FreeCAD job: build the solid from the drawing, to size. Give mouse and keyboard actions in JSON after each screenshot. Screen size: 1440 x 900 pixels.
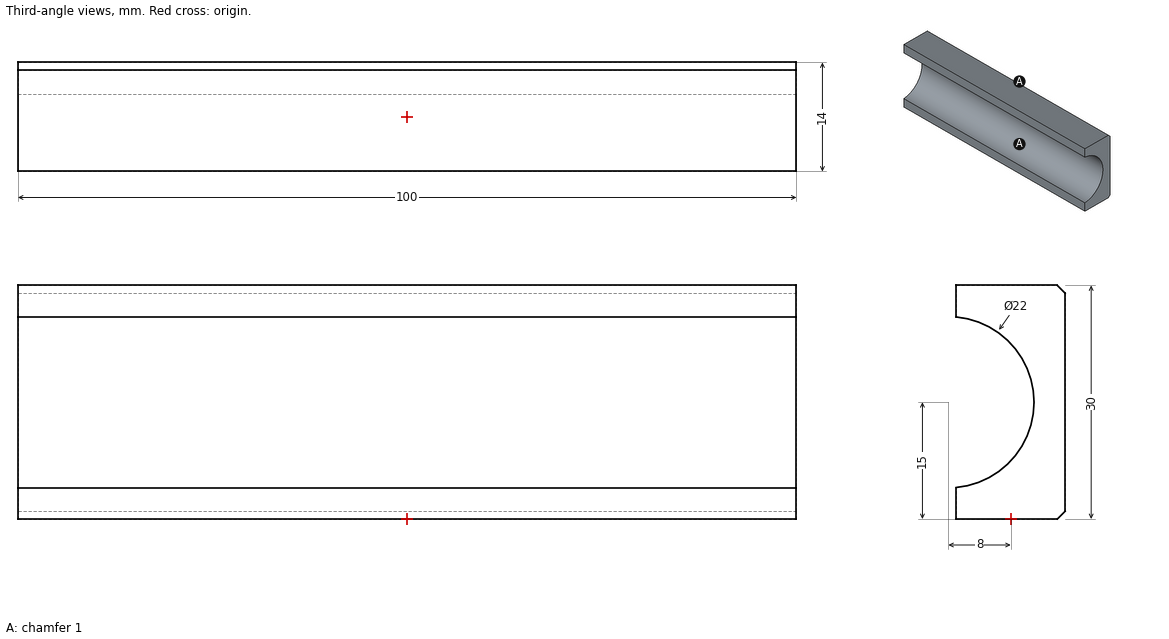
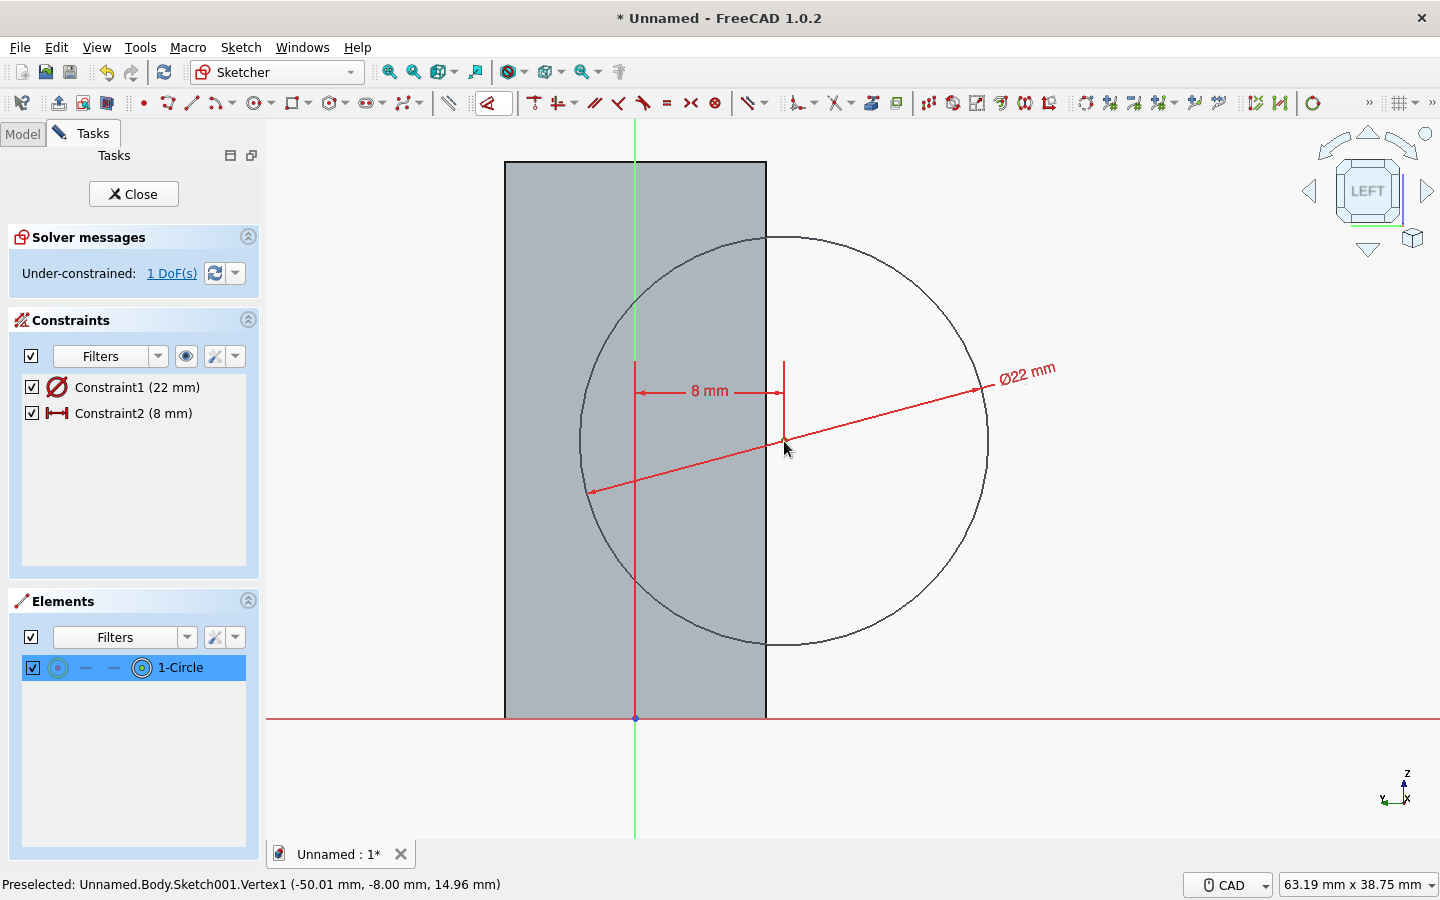
{"action": "key", "text": "i"}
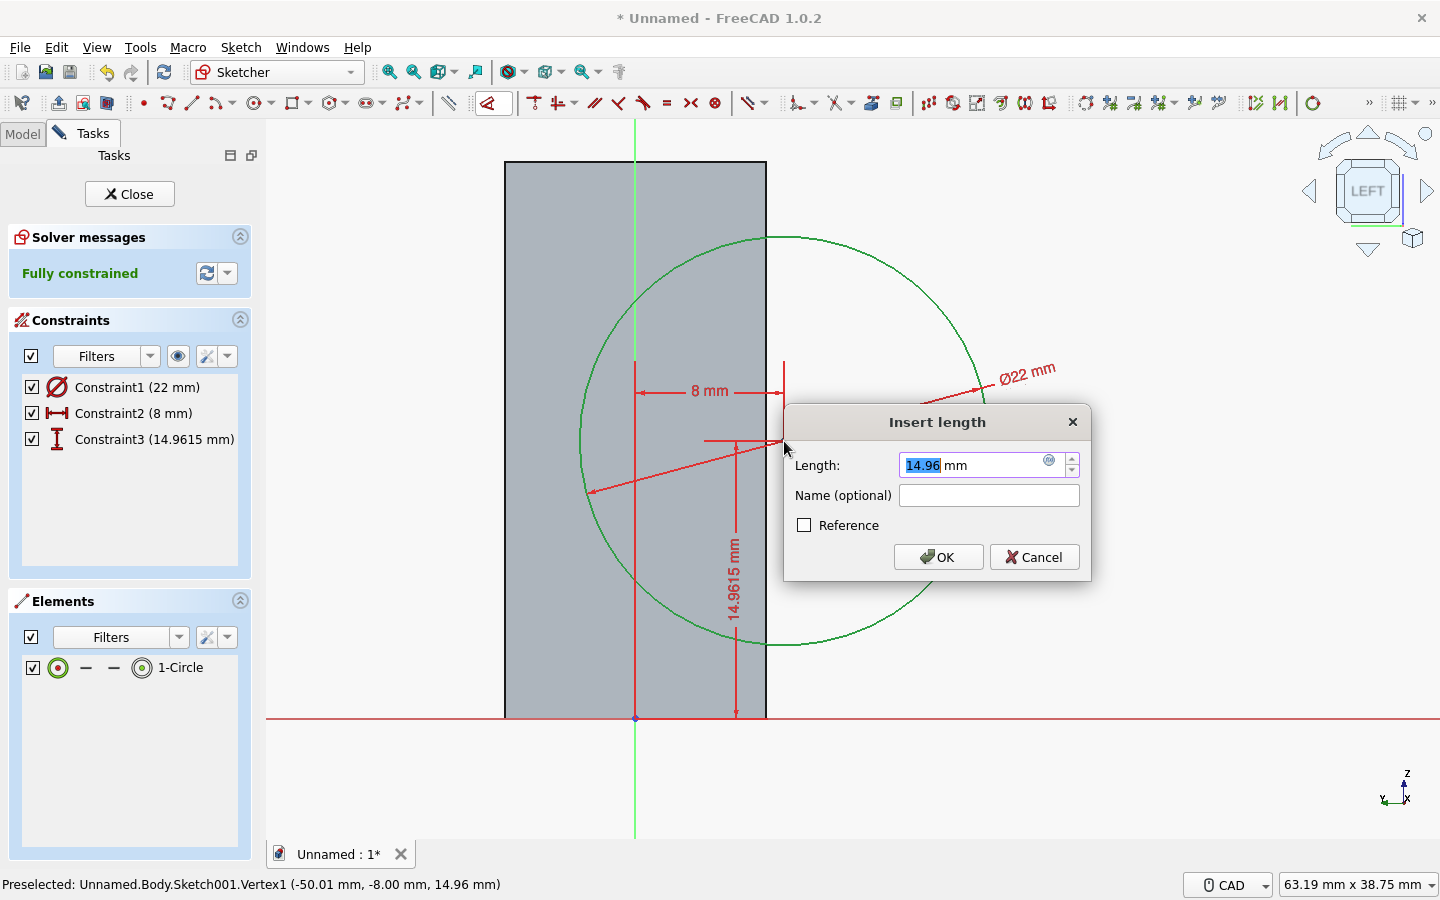
{"action": "type", "text": "15"}
{"action": "key", "text": "Return"}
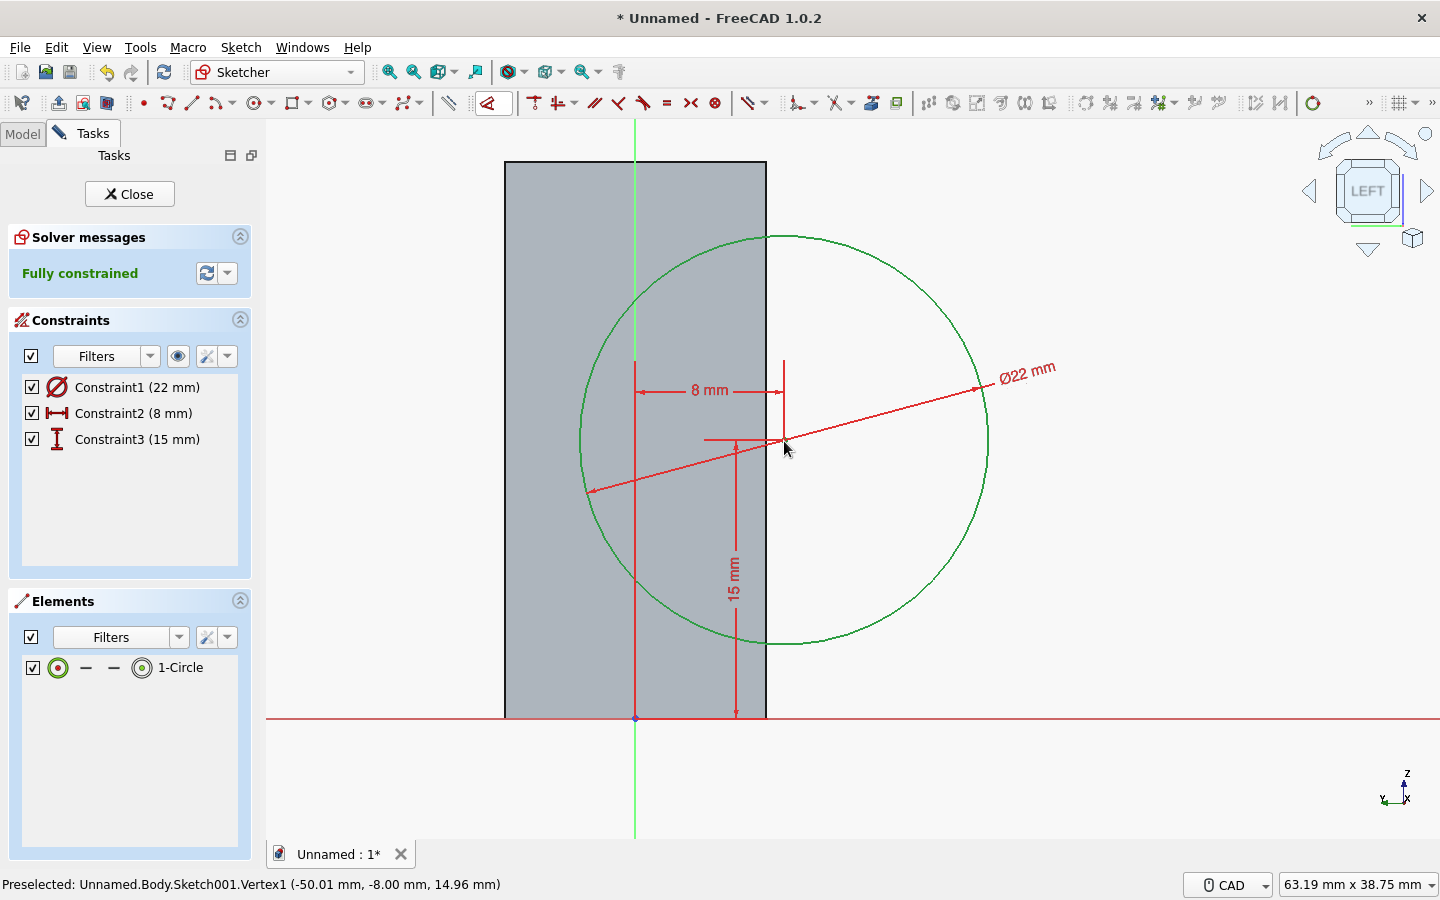
{"action": "left_click", "coordinate": [130, 194]}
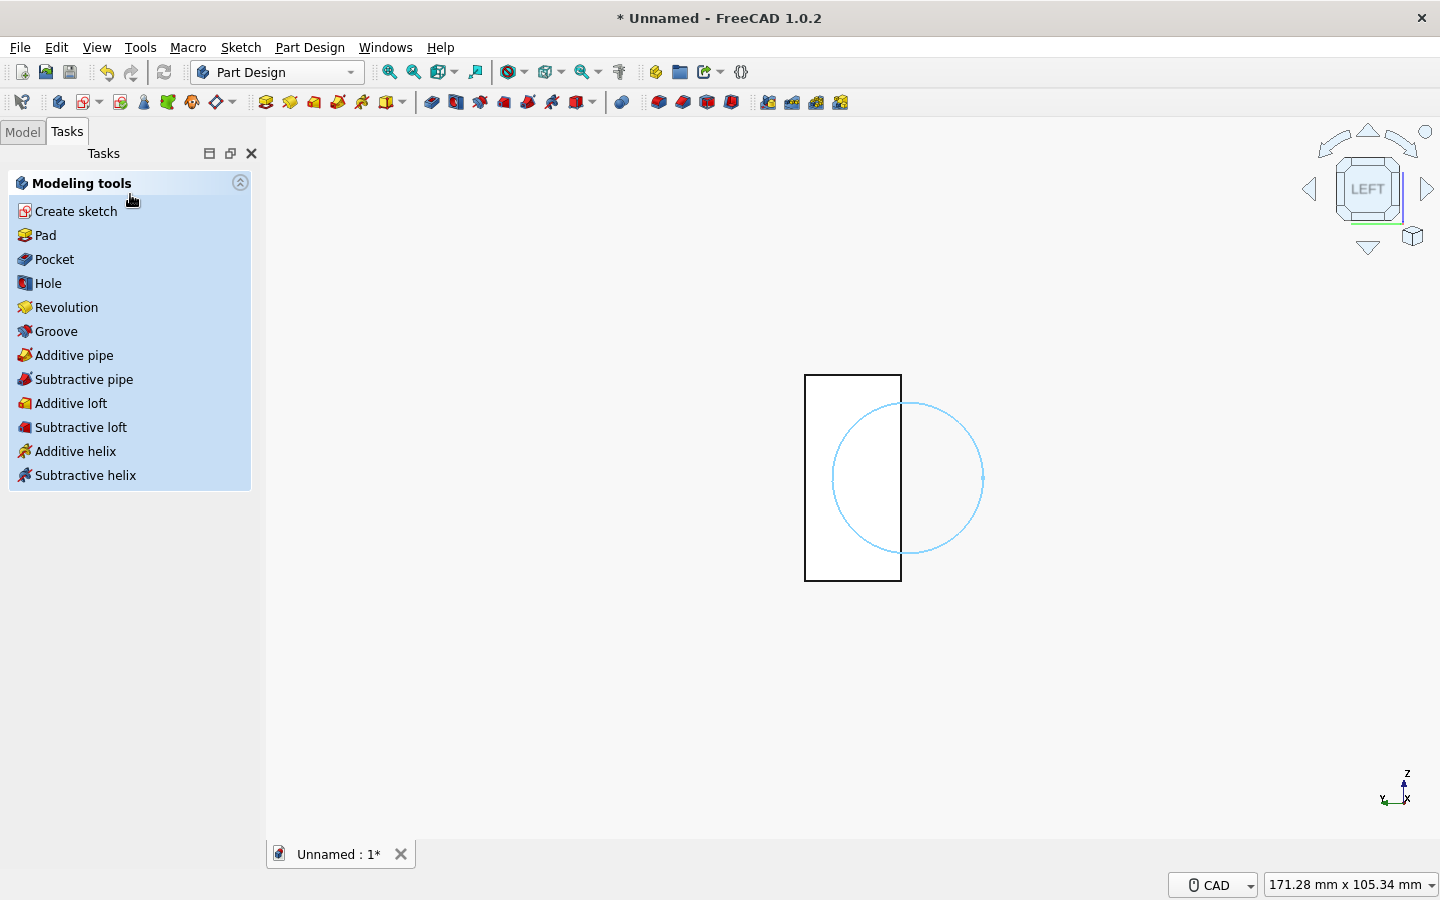
{"action": "left_click", "coordinate": [432, 102]}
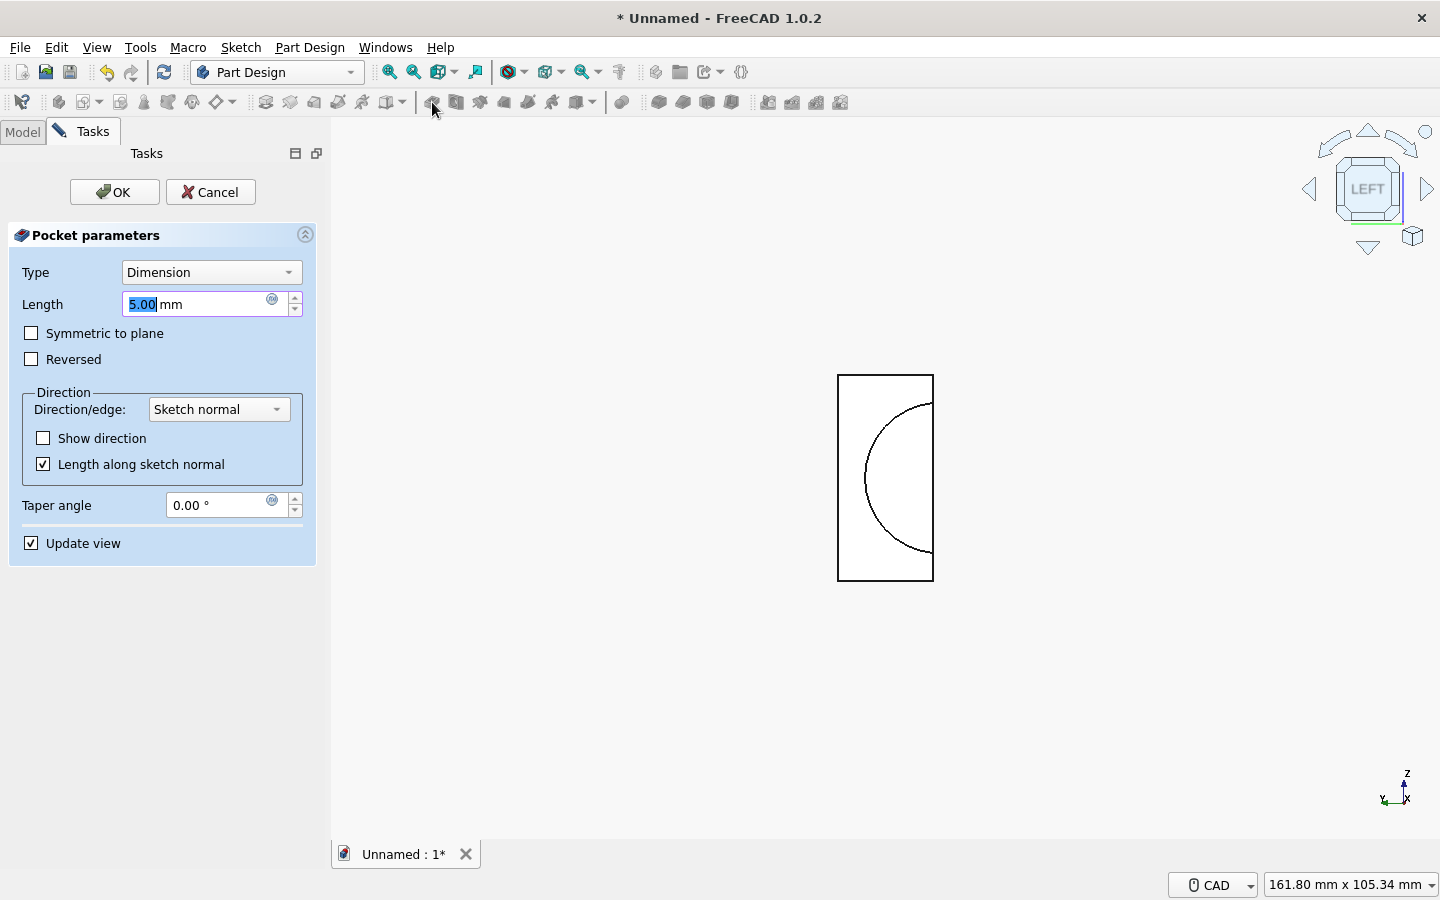
{"action": "left_click", "coordinate": [212, 272]}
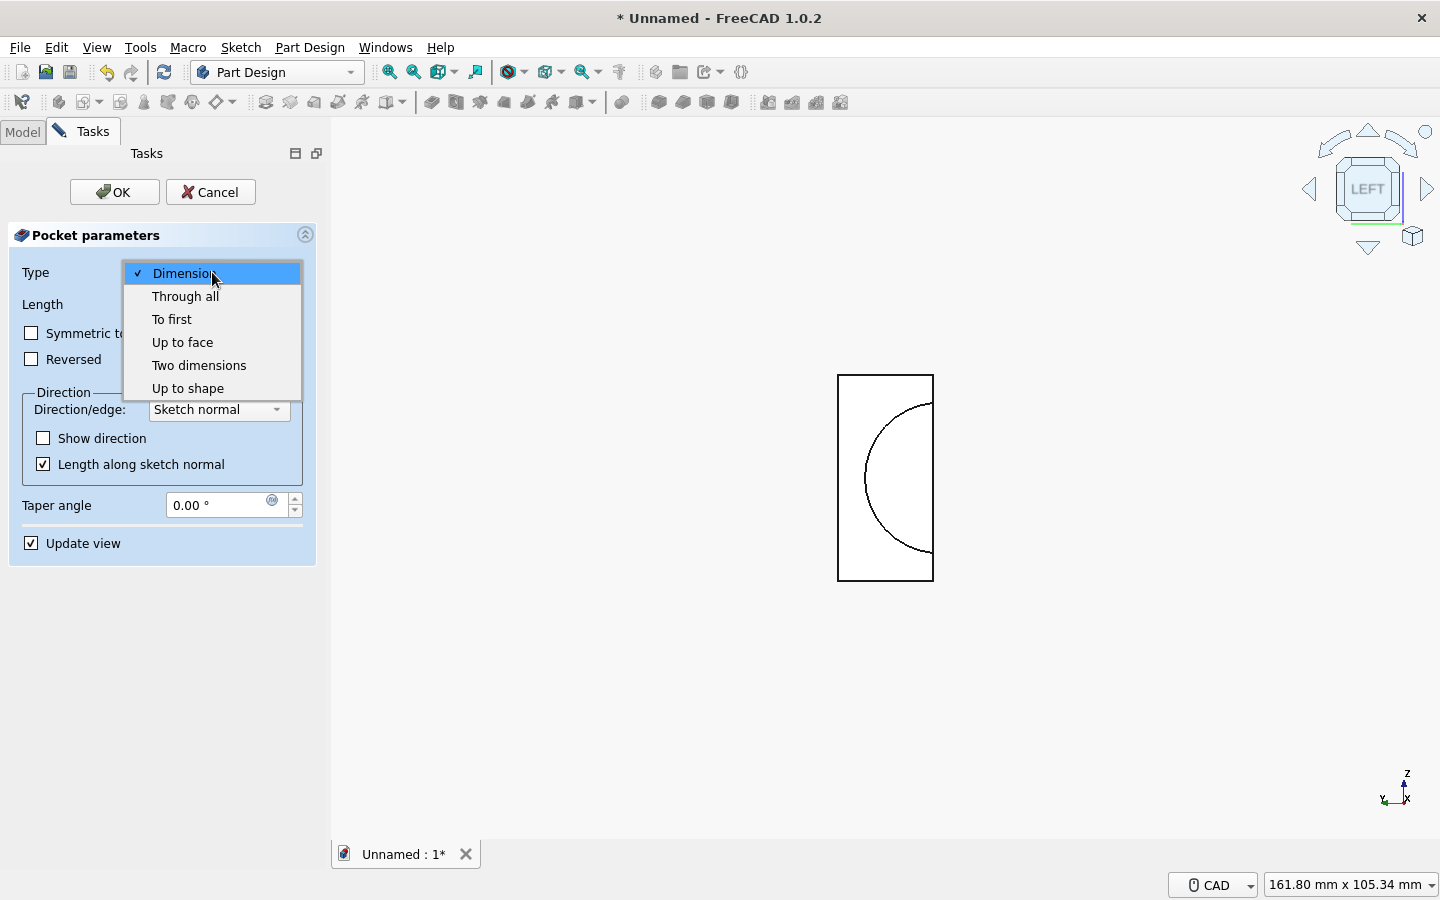
{"action": "left_click", "coordinate": [212, 296]}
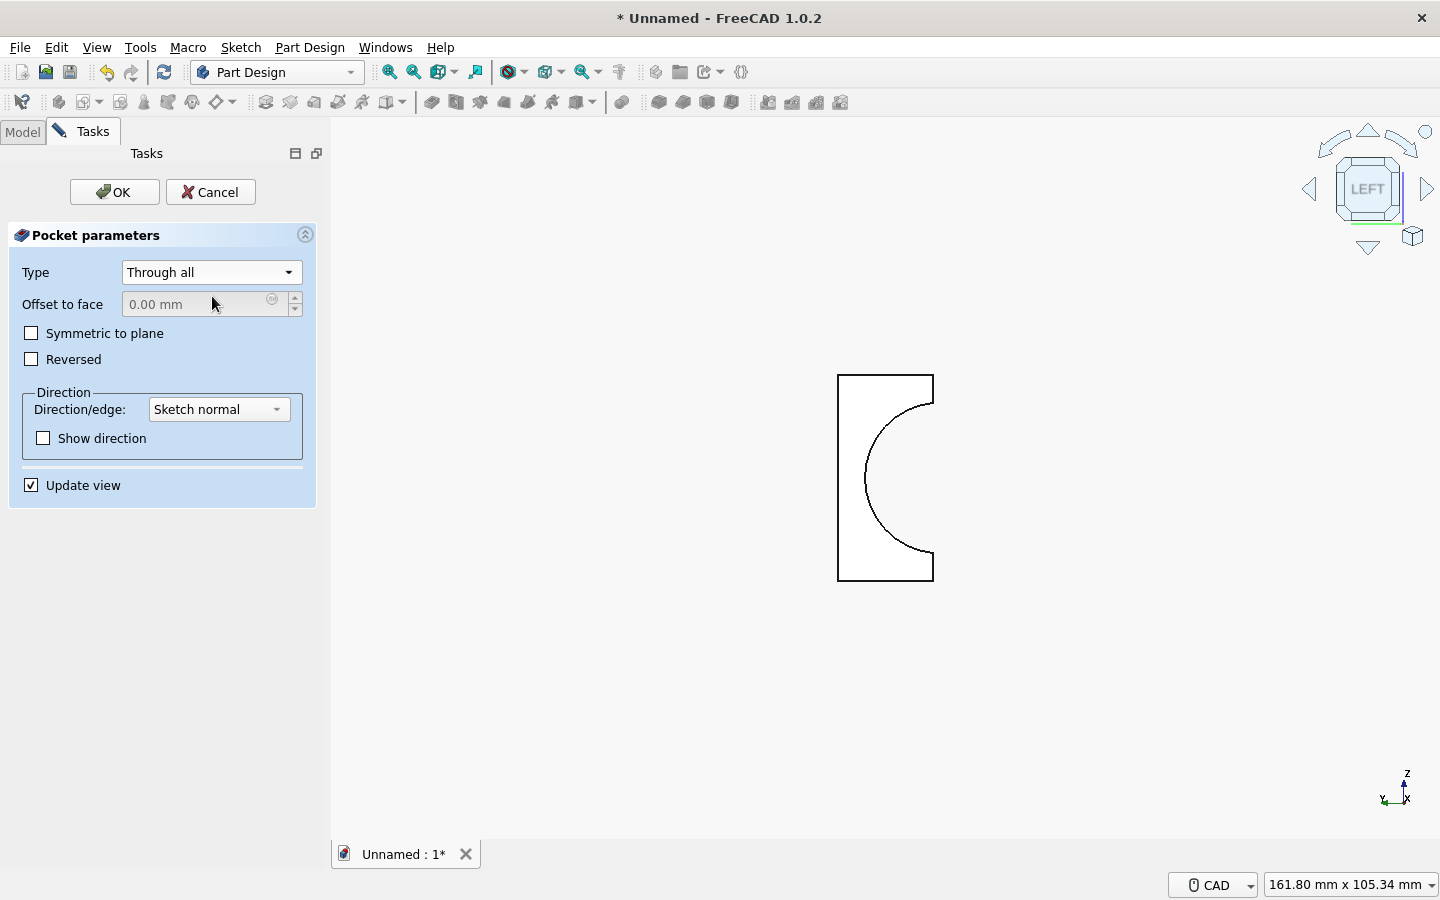
{"action": "left_click", "coordinate": [115, 192]}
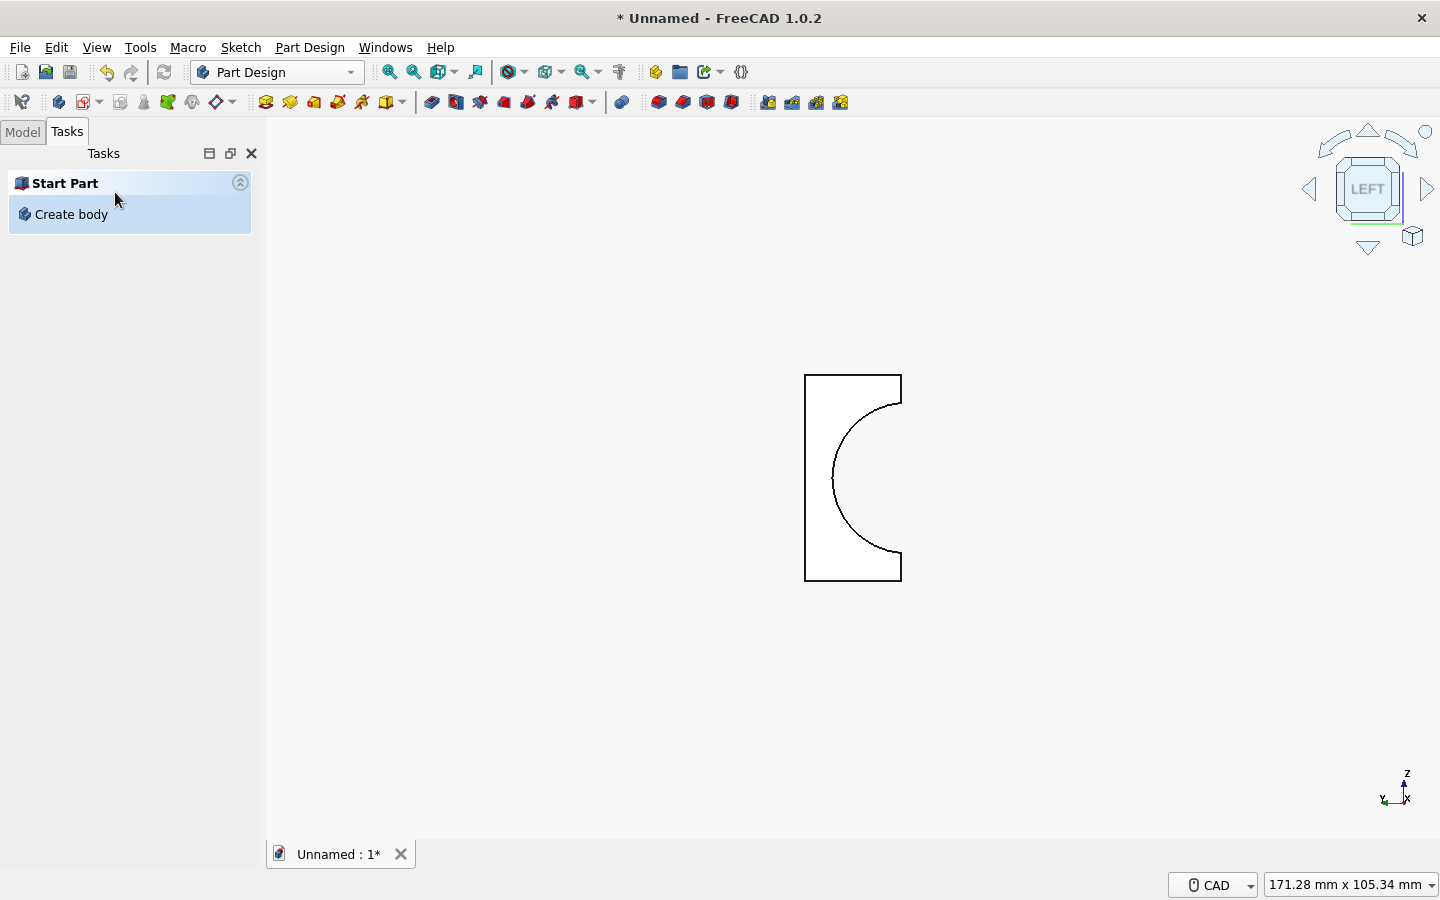
{"action": "left_click", "coordinate": [390, 72]}